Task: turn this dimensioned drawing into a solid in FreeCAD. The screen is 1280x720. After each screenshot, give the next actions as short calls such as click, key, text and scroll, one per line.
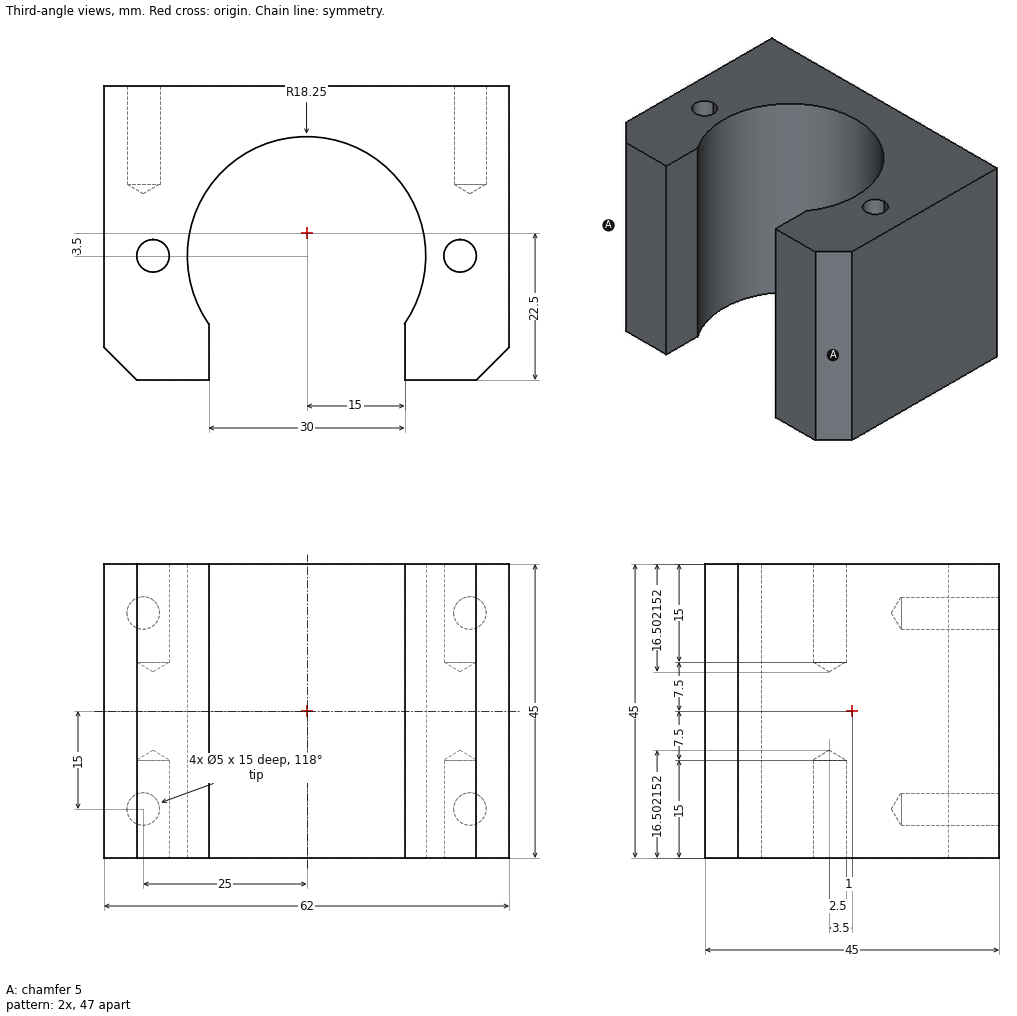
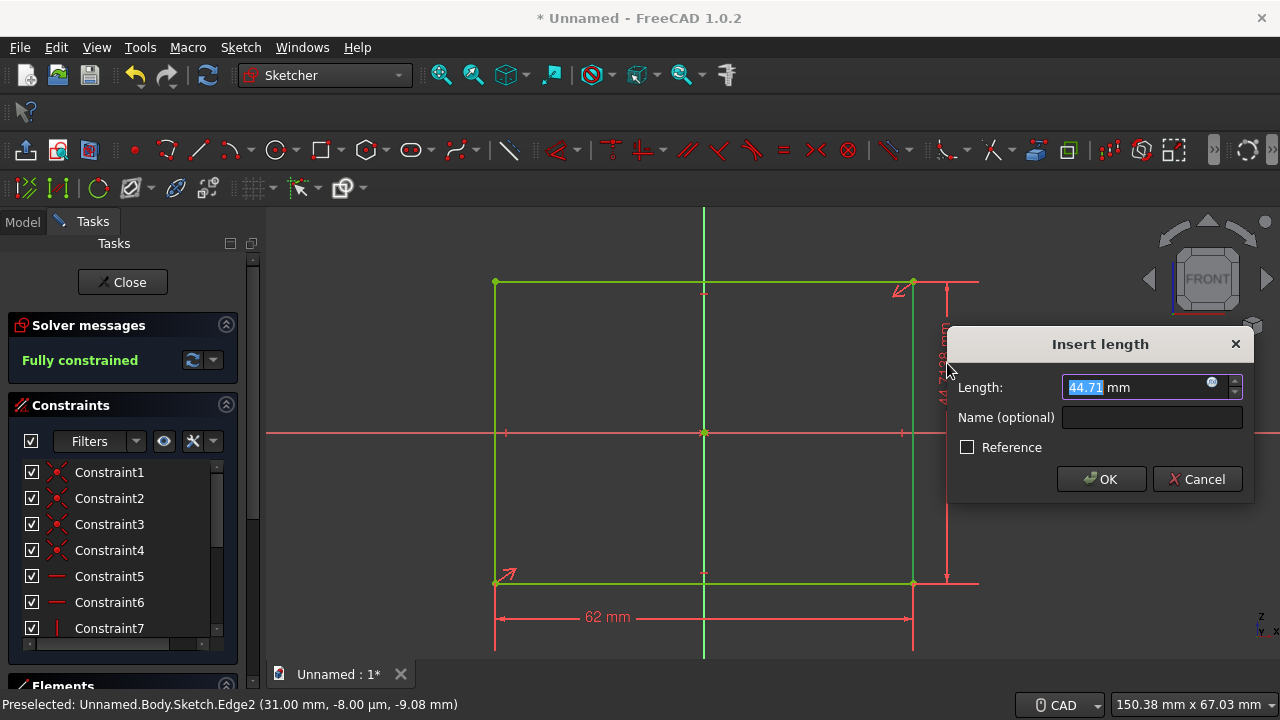
text(45)
key(Return)
key(Escape)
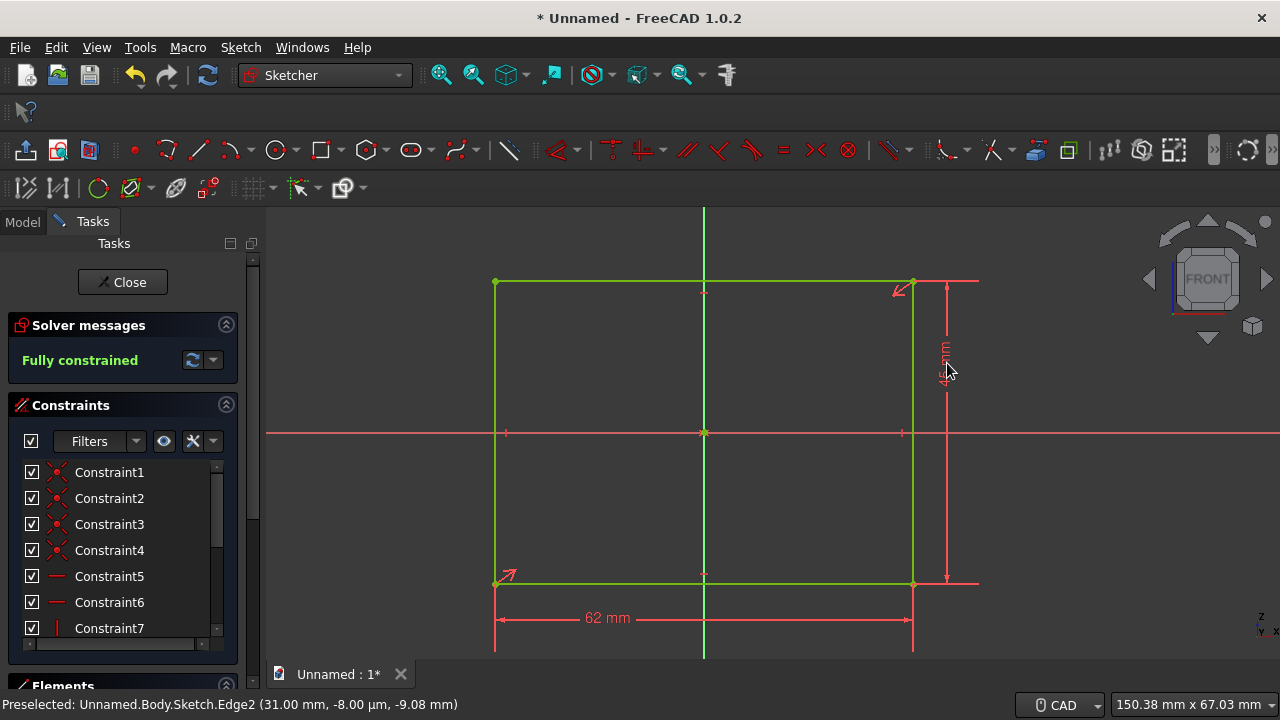
click(123, 282)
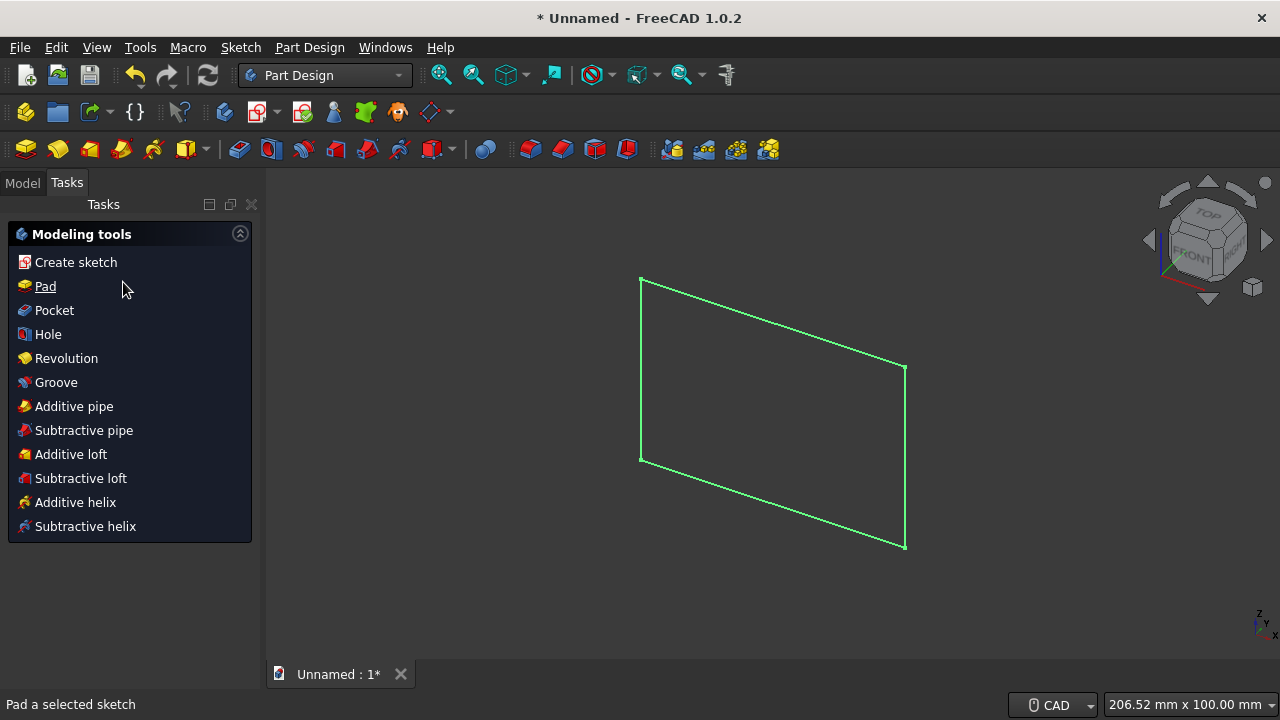
click(26, 150)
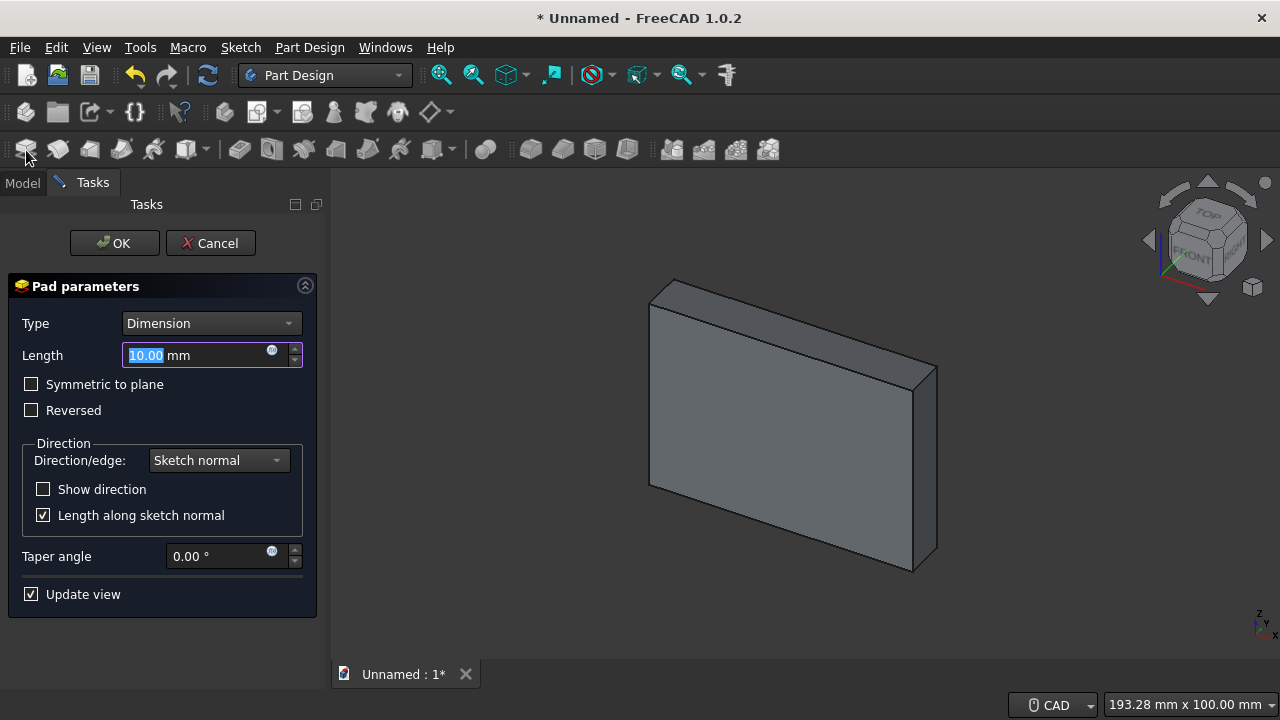
text(45)
key(Tab)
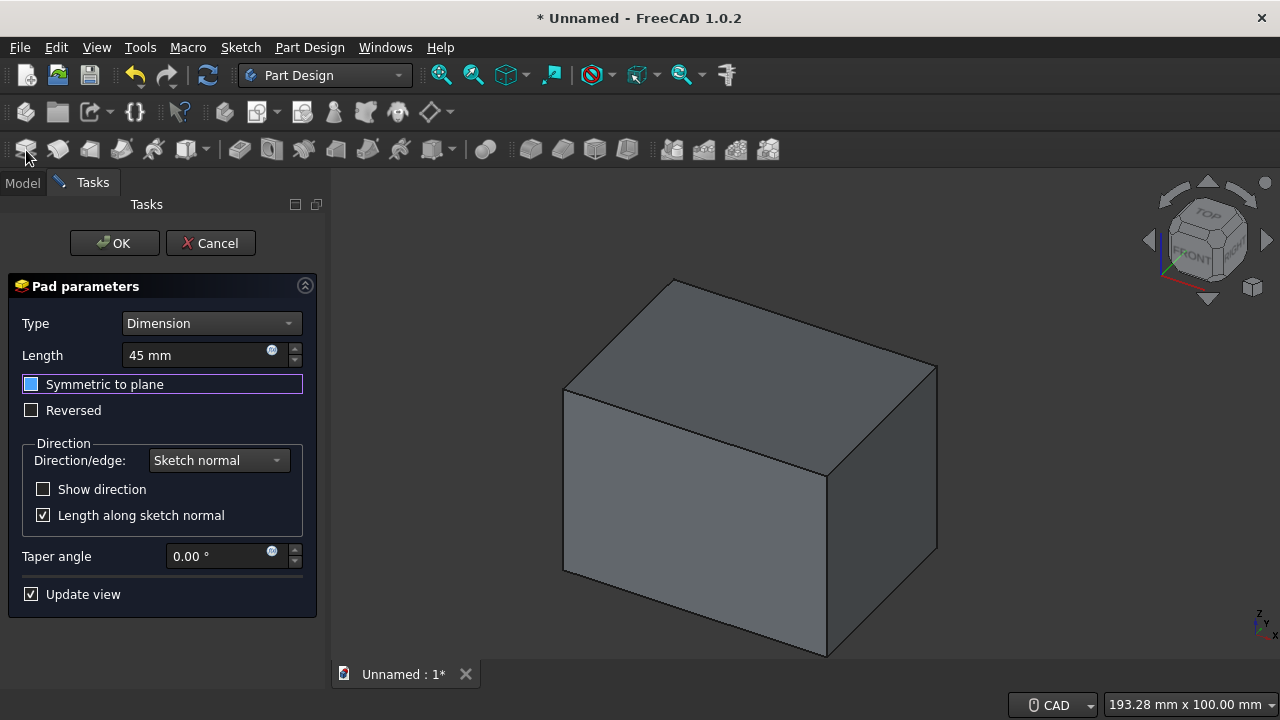
click(30, 384)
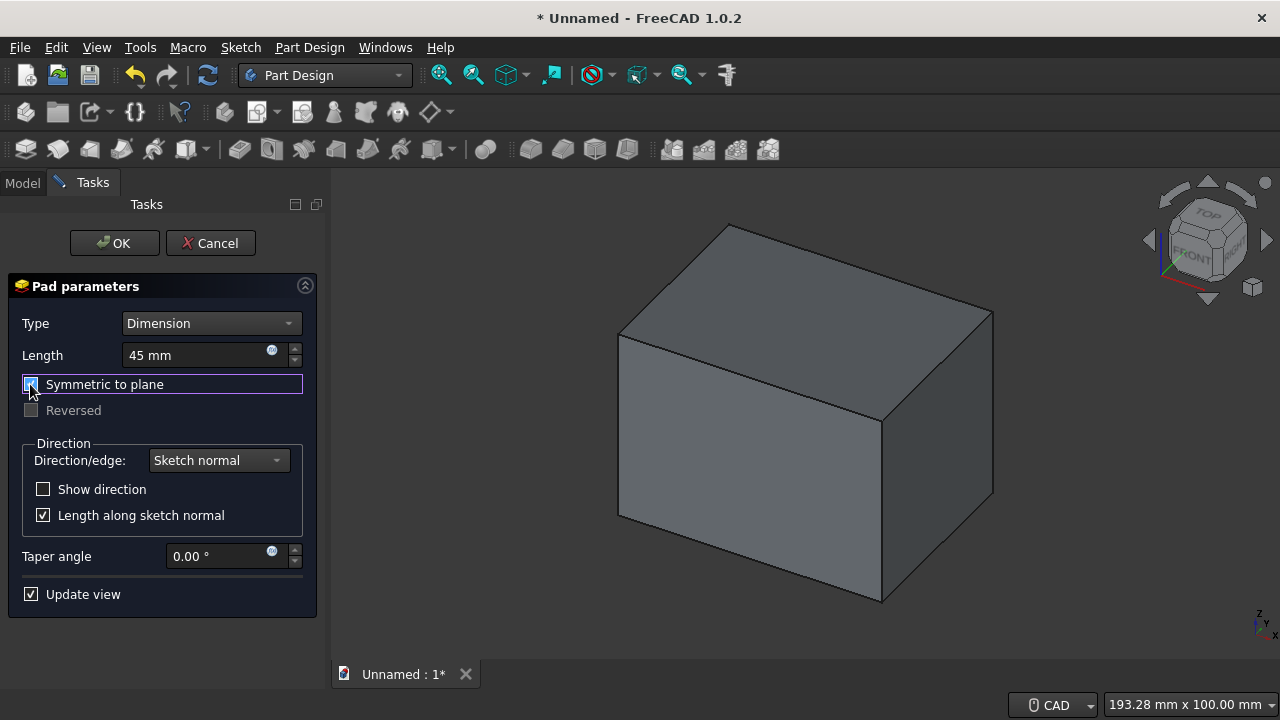
click(115, 243)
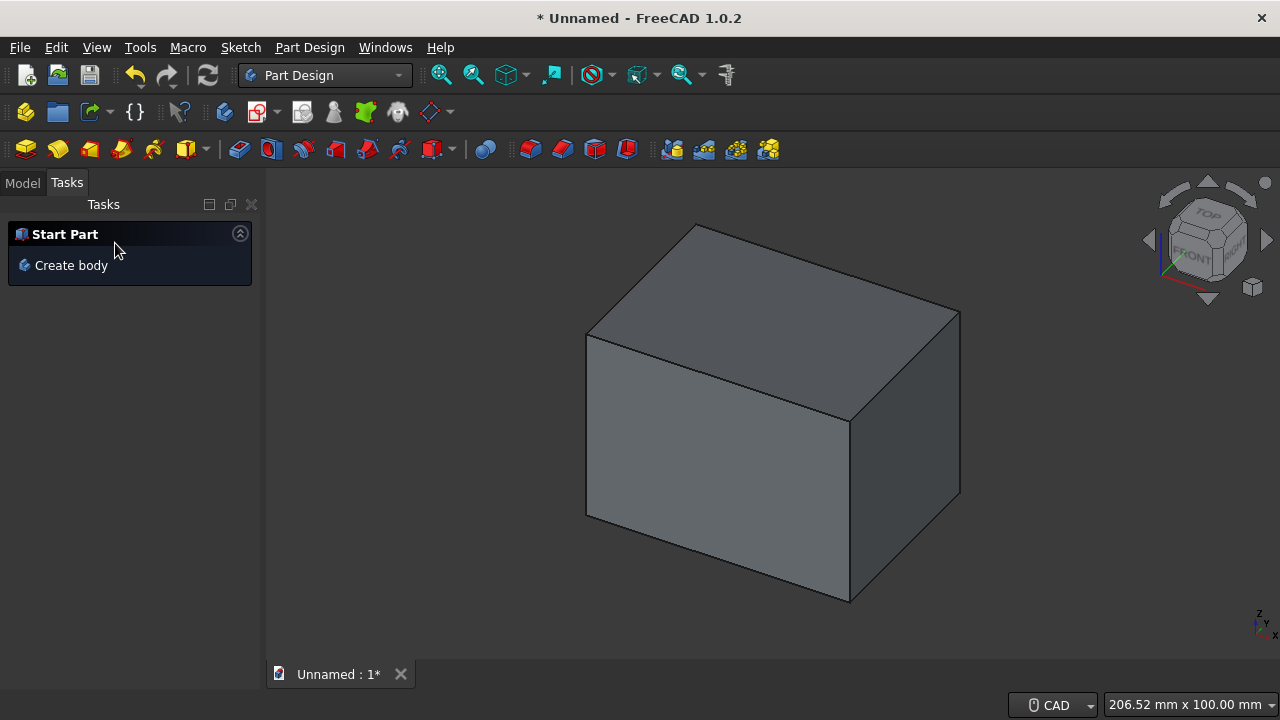
key(5)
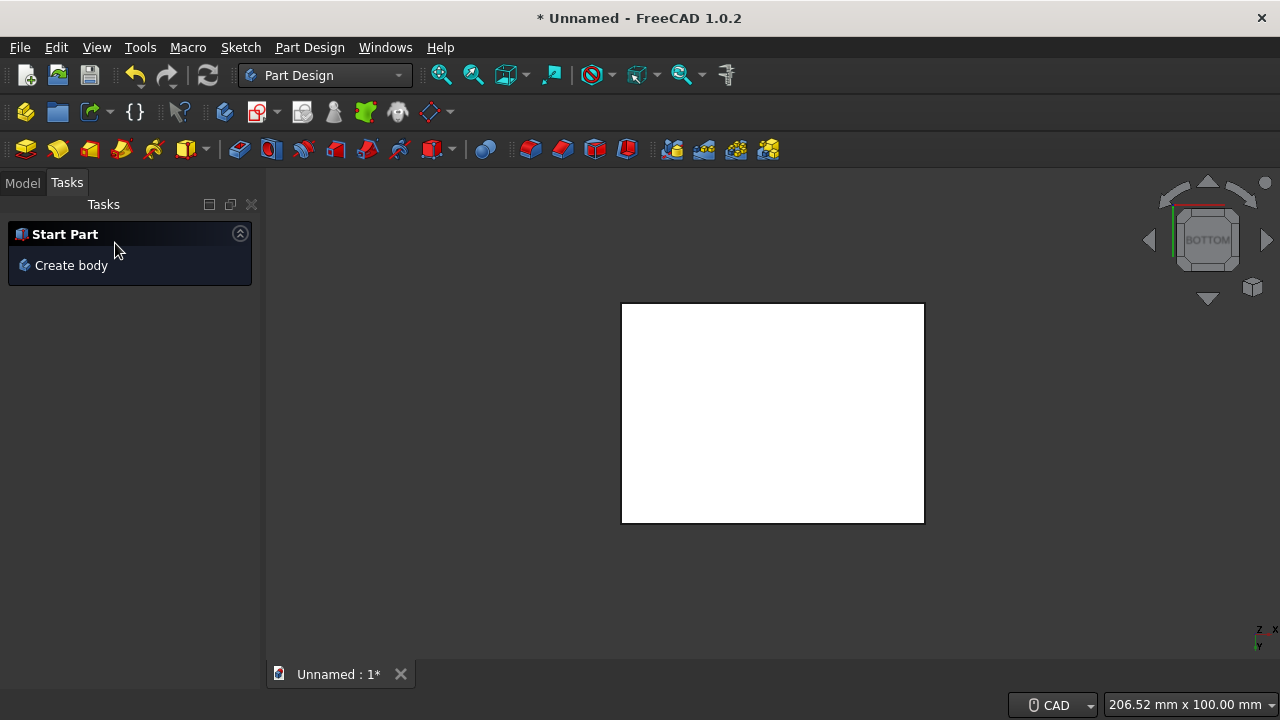
click(773, 412)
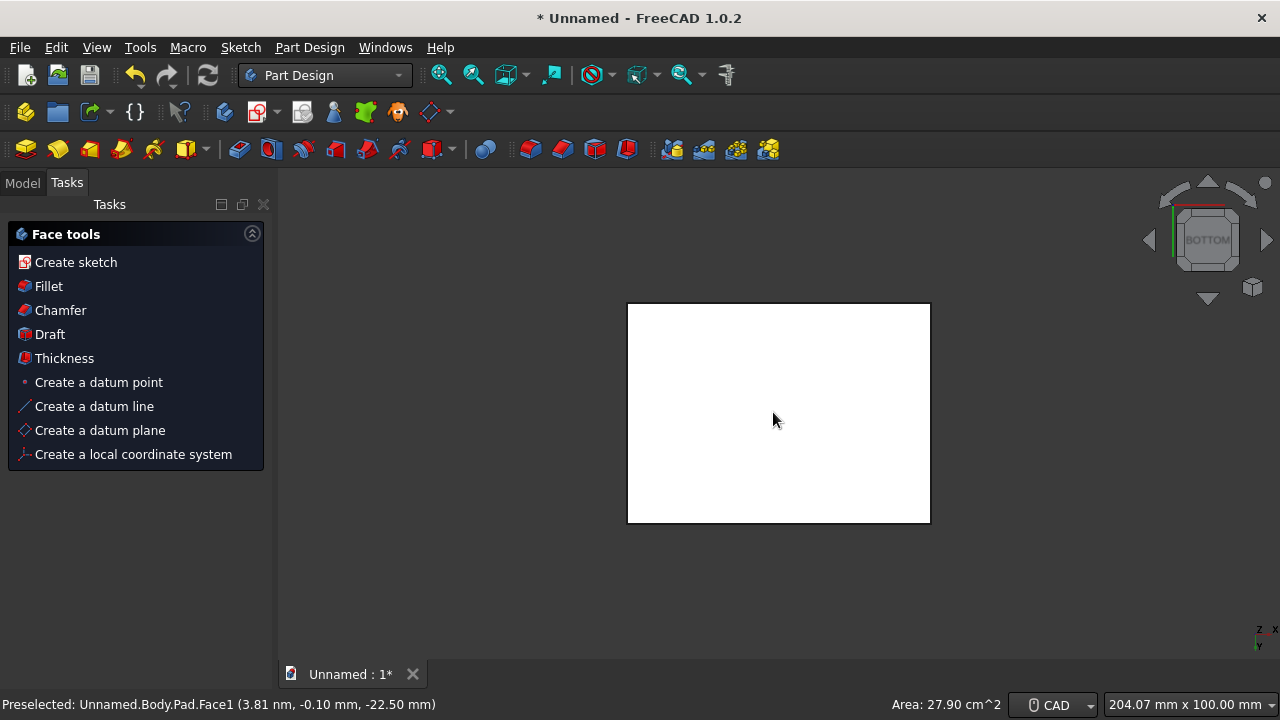
click(258, 112)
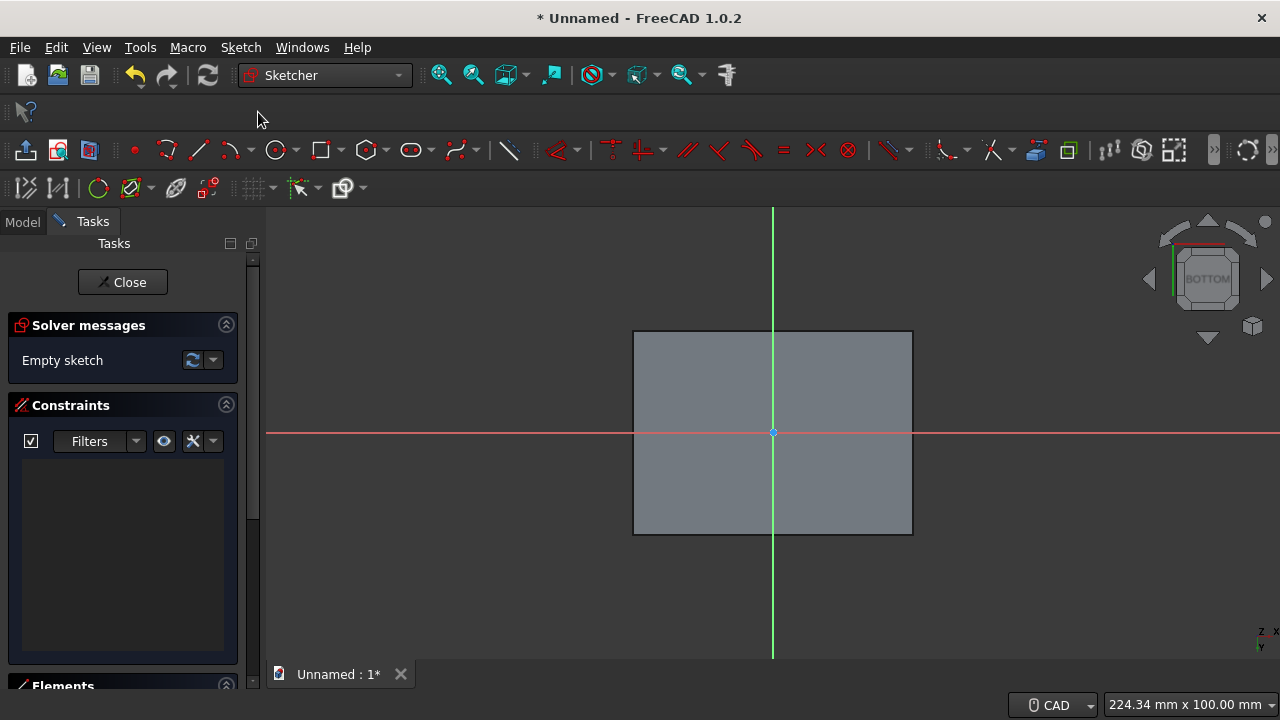
scroll(856, 394, up, 3)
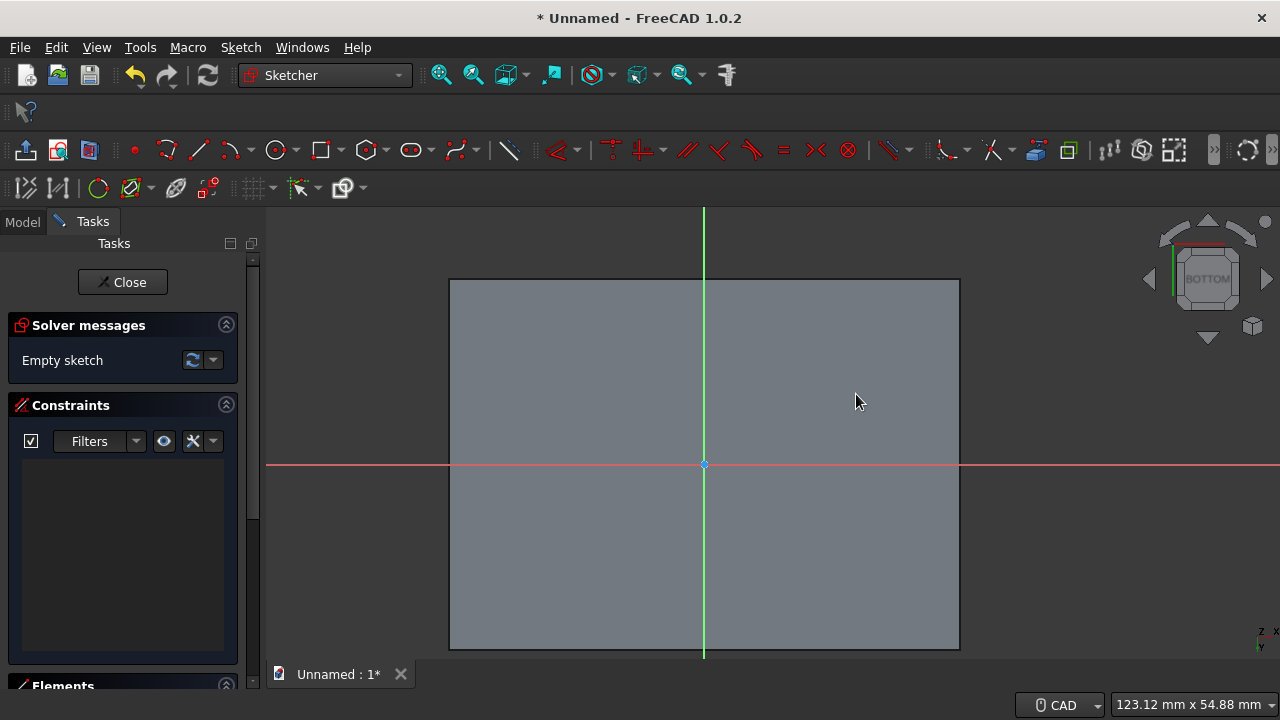
click(168, 150)